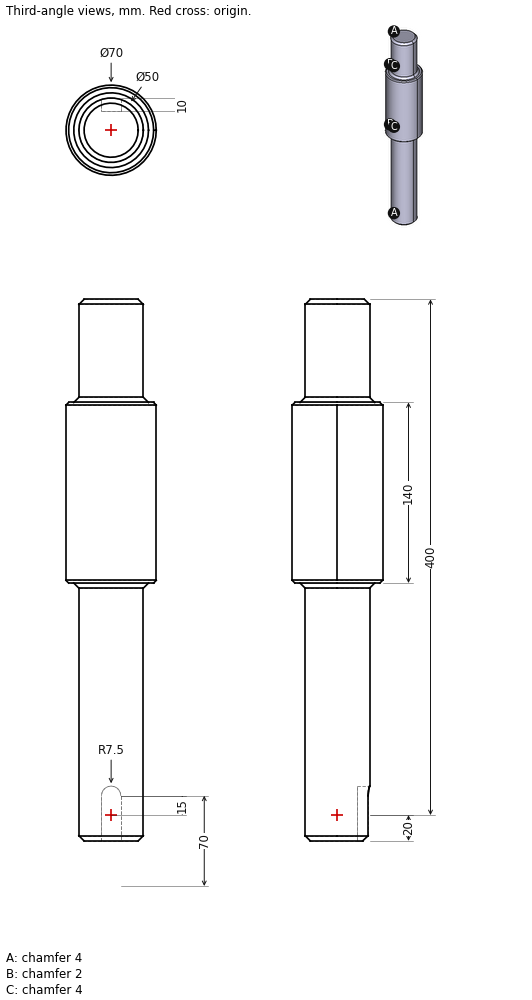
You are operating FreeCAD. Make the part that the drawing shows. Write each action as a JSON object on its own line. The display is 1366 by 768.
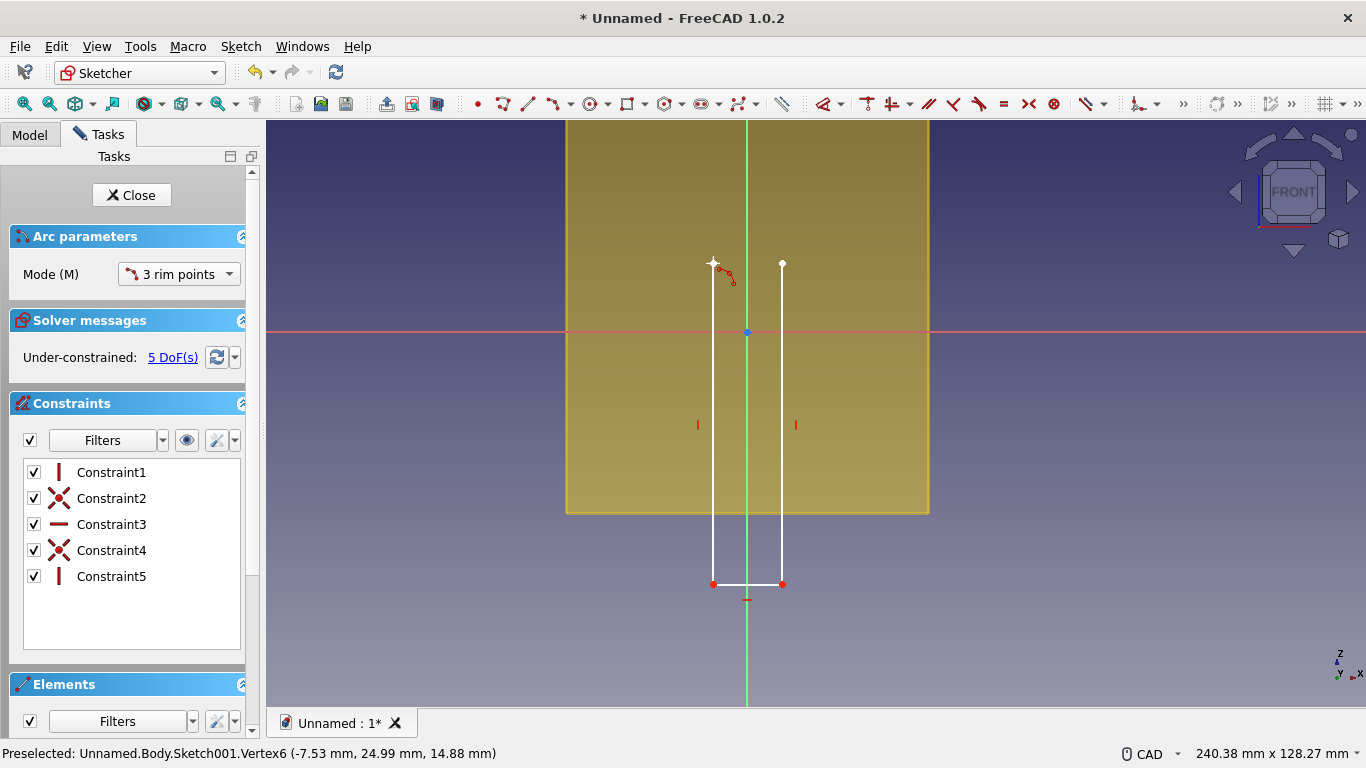
{"action": "left_click", "coordinate": [713, 264]}
{"action": "left_click", "coordinate": [782, 264]}
{"action": "left_click", "coordinate": [768, 236]}
{"action": "key", "text": "Escape"}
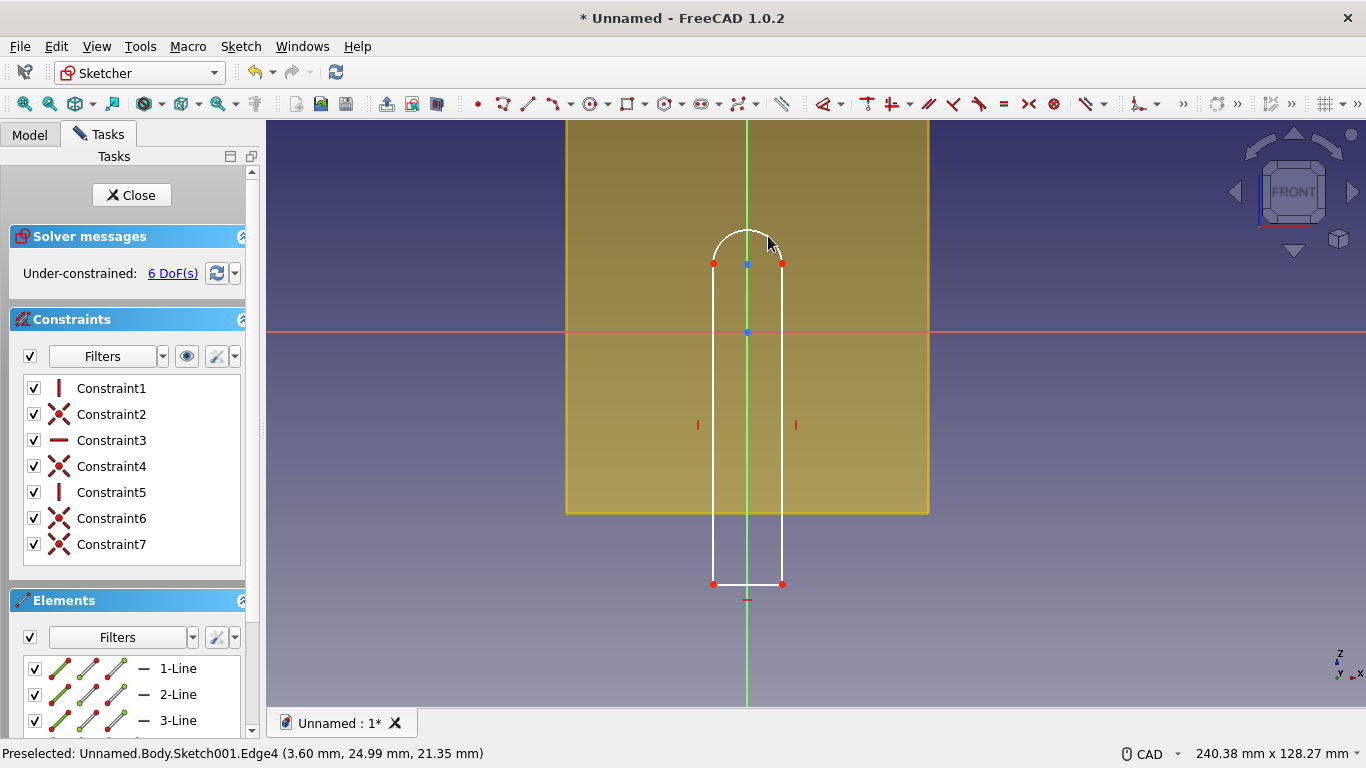
{"action": "left_click", "coordinate": [782, 360]}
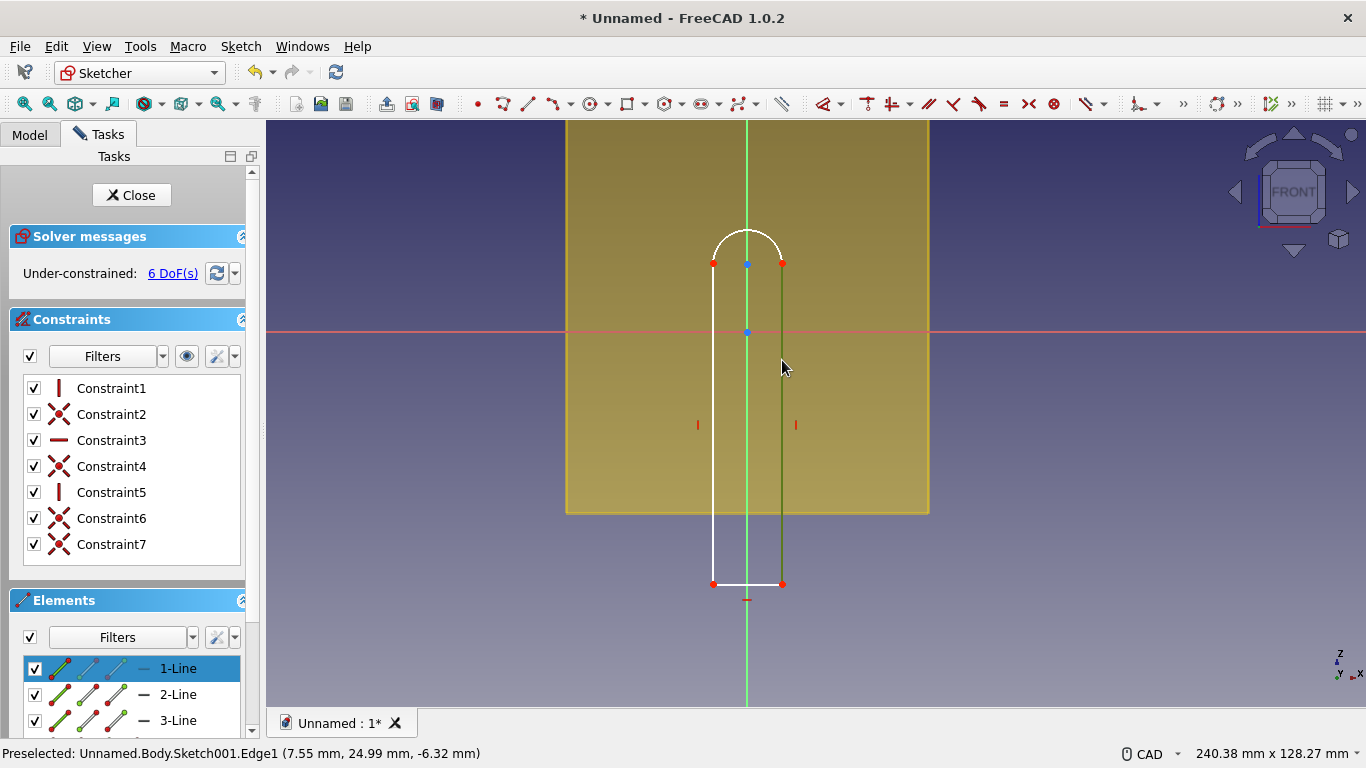
{"action": "left_click", "coordinate": [768, 237]}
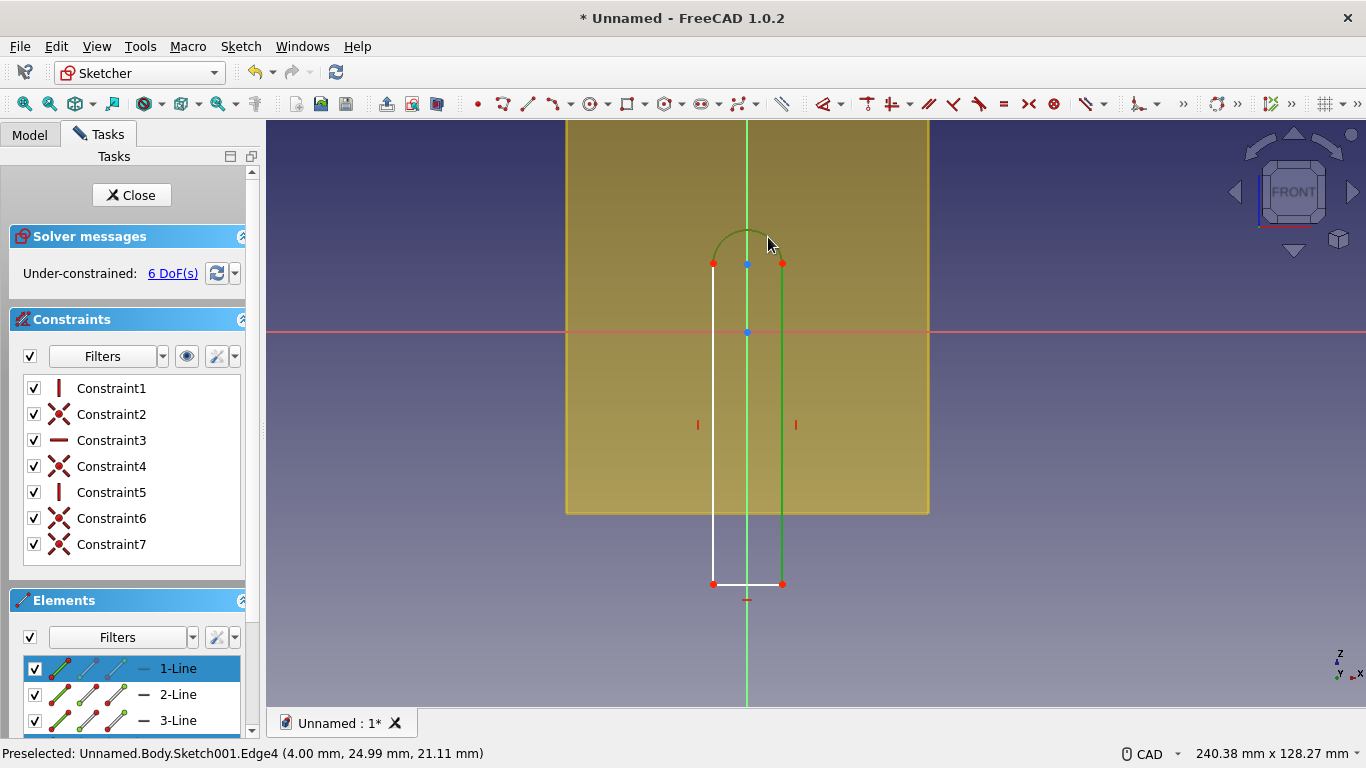
{"action": "left_click", "coordinate": [979, 104]}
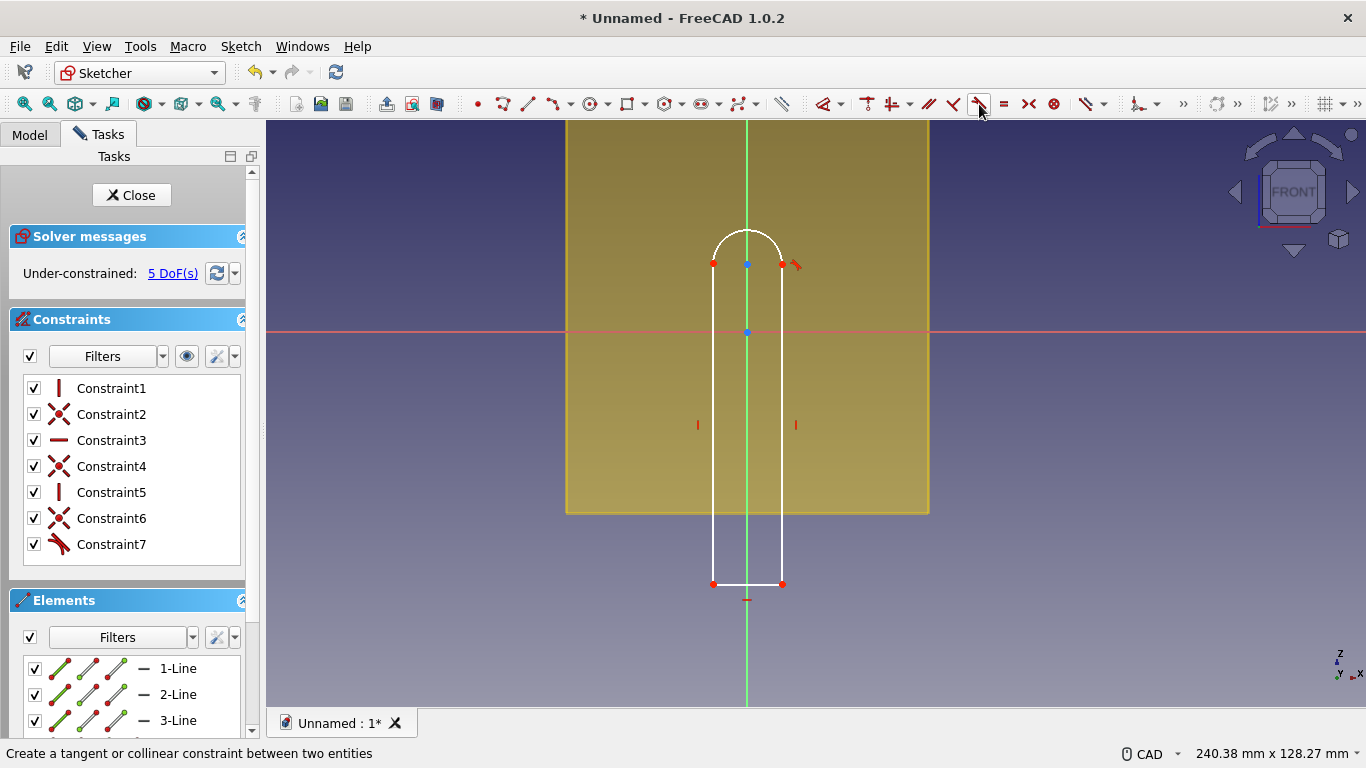
{"action": "left_click", "coordinate": [713, 489]}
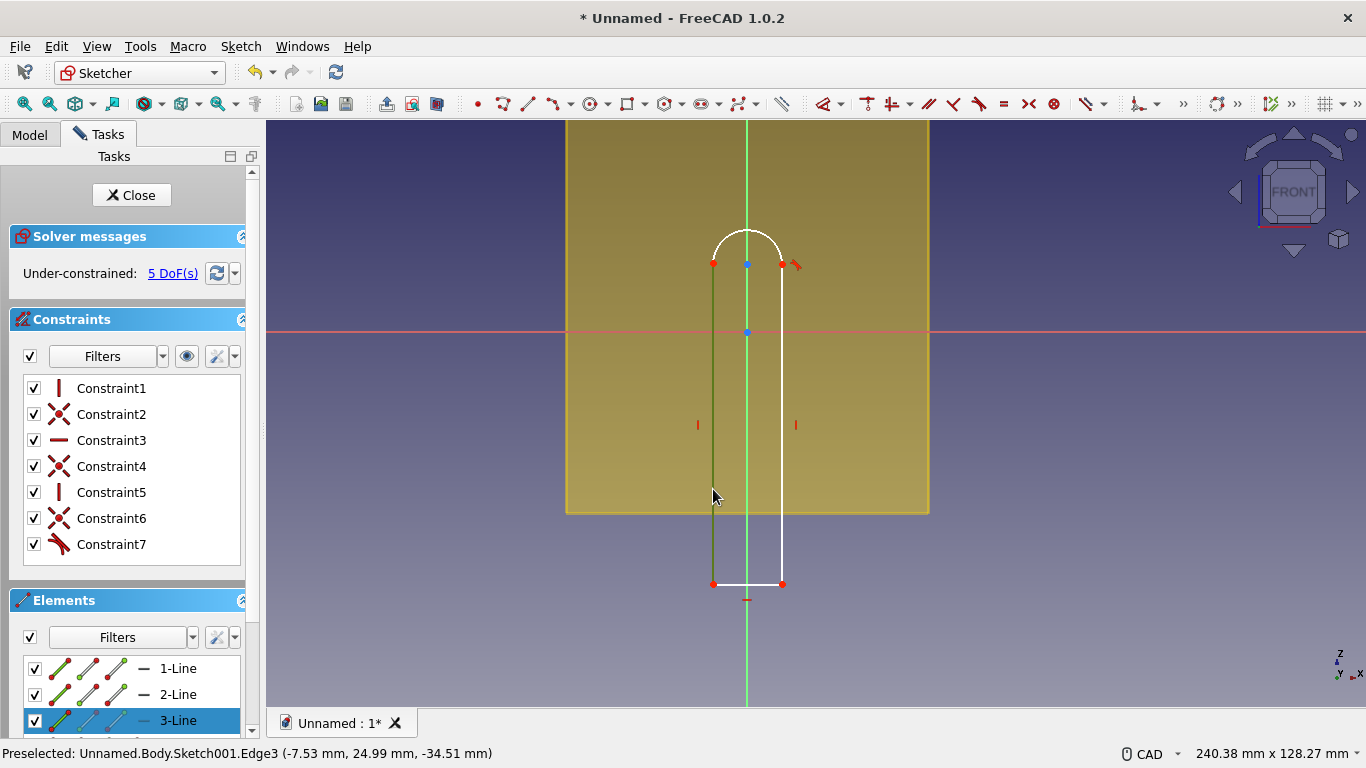
{"action": "left_click", "coordinate": [768, 237]}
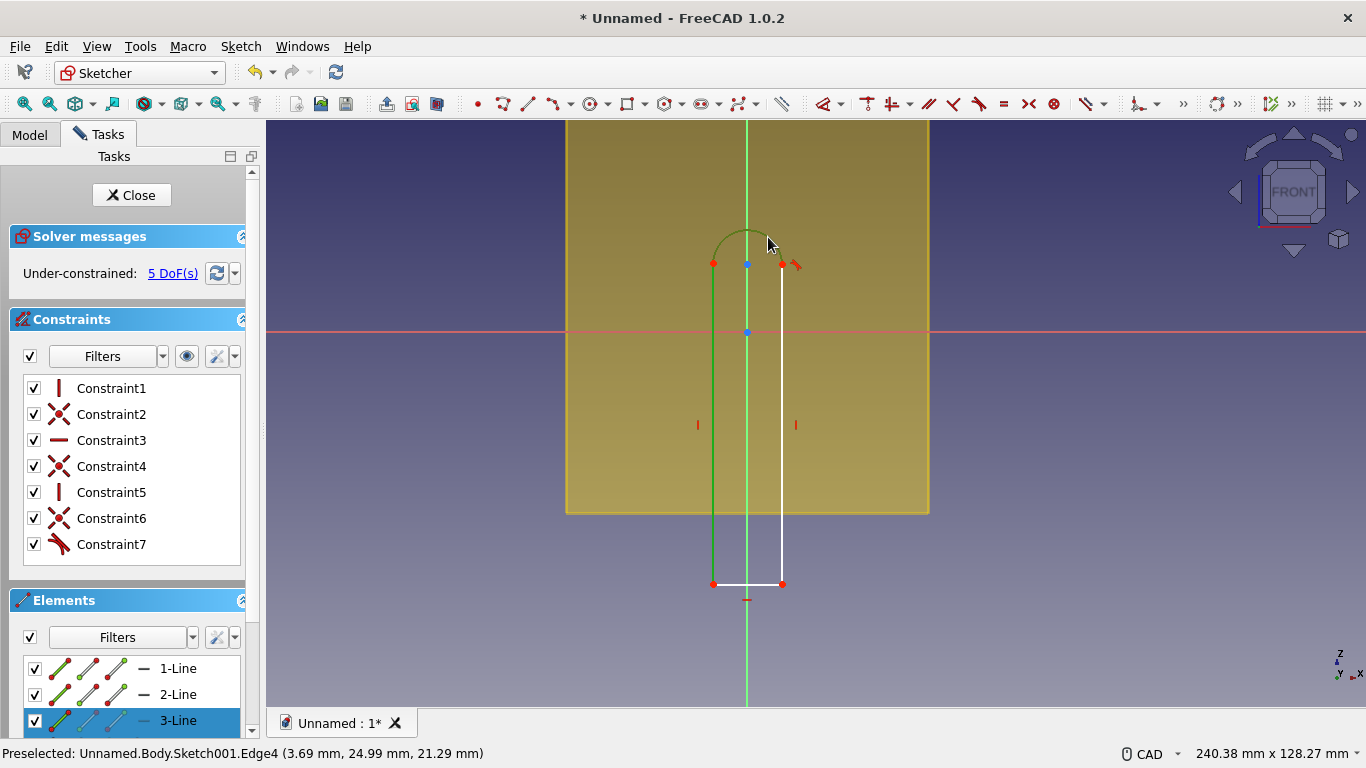
{"action": "left_click", "coordinate": [979, 104]}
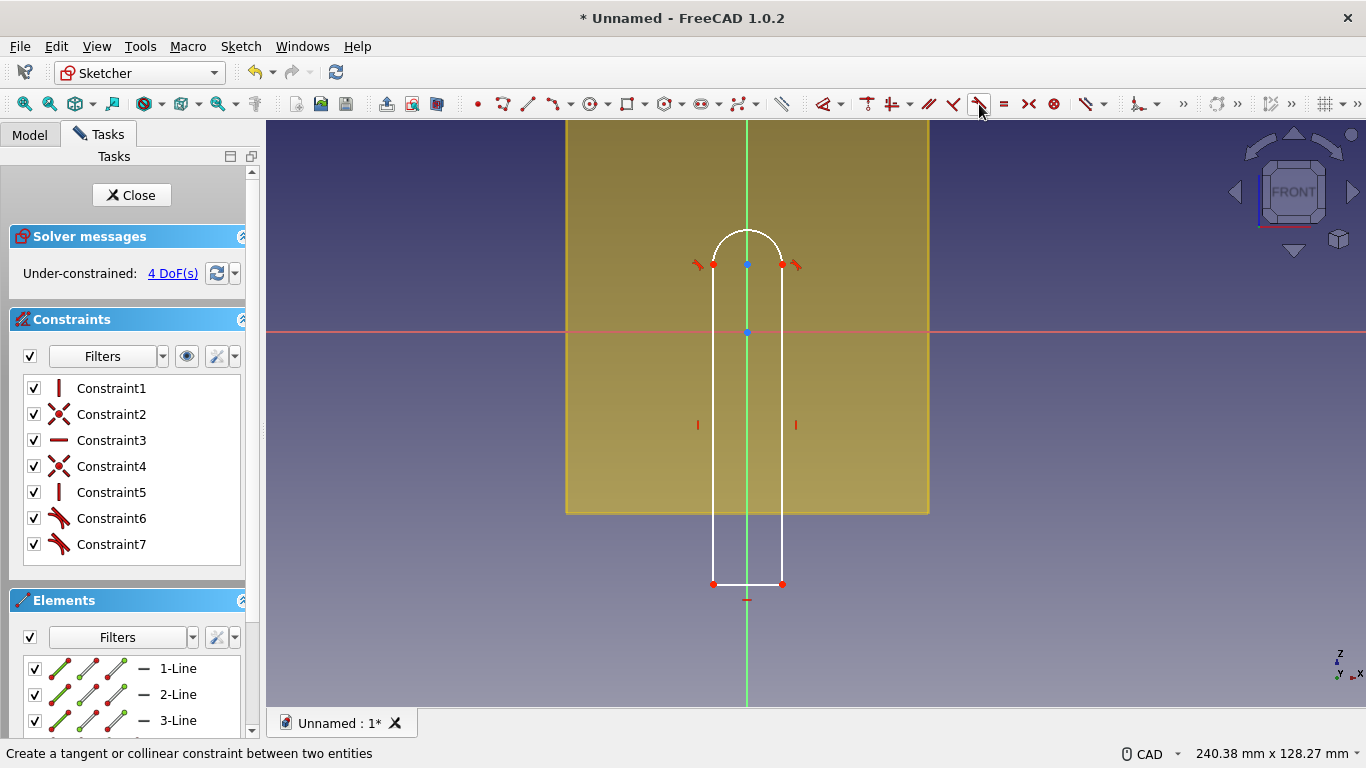
{"action": "left_click", "coordinate": [747, 265]}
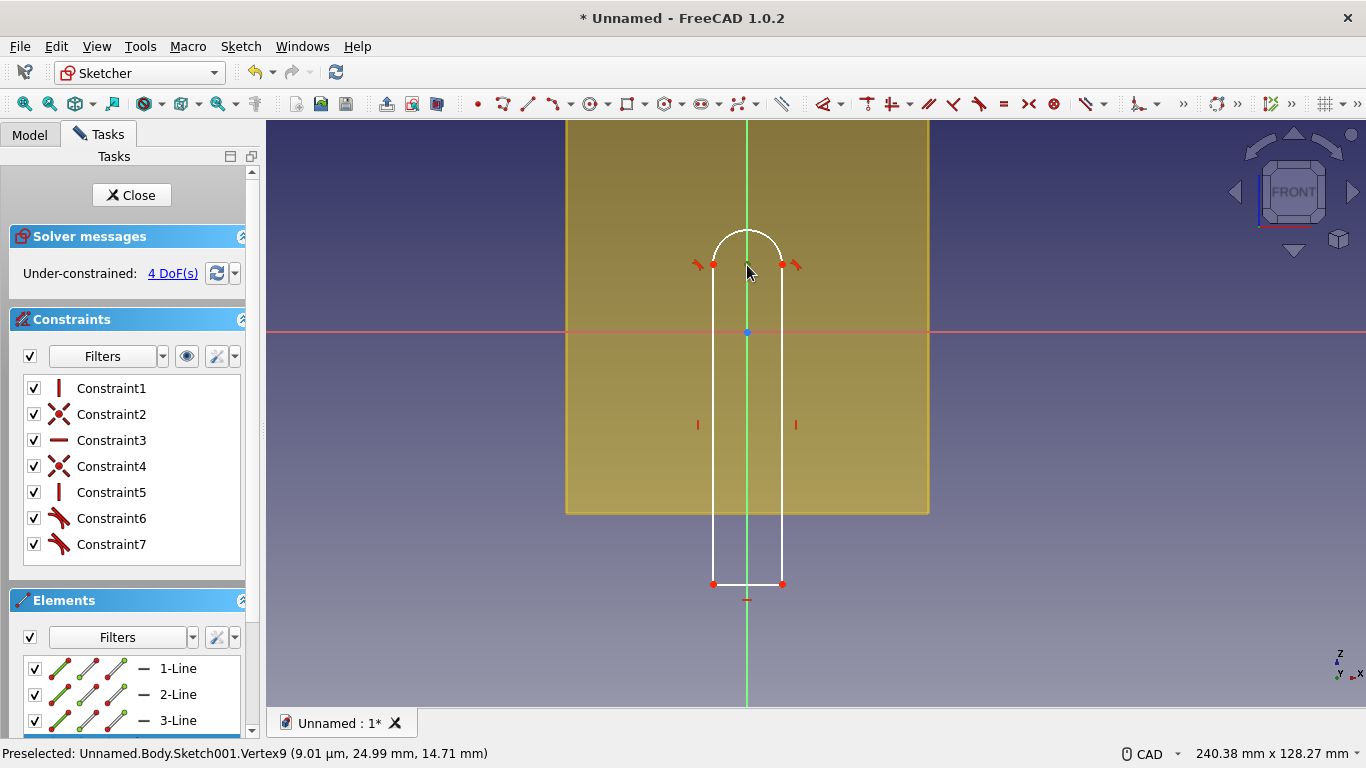
{"action": "left_click", "coordinate": [747, 641]}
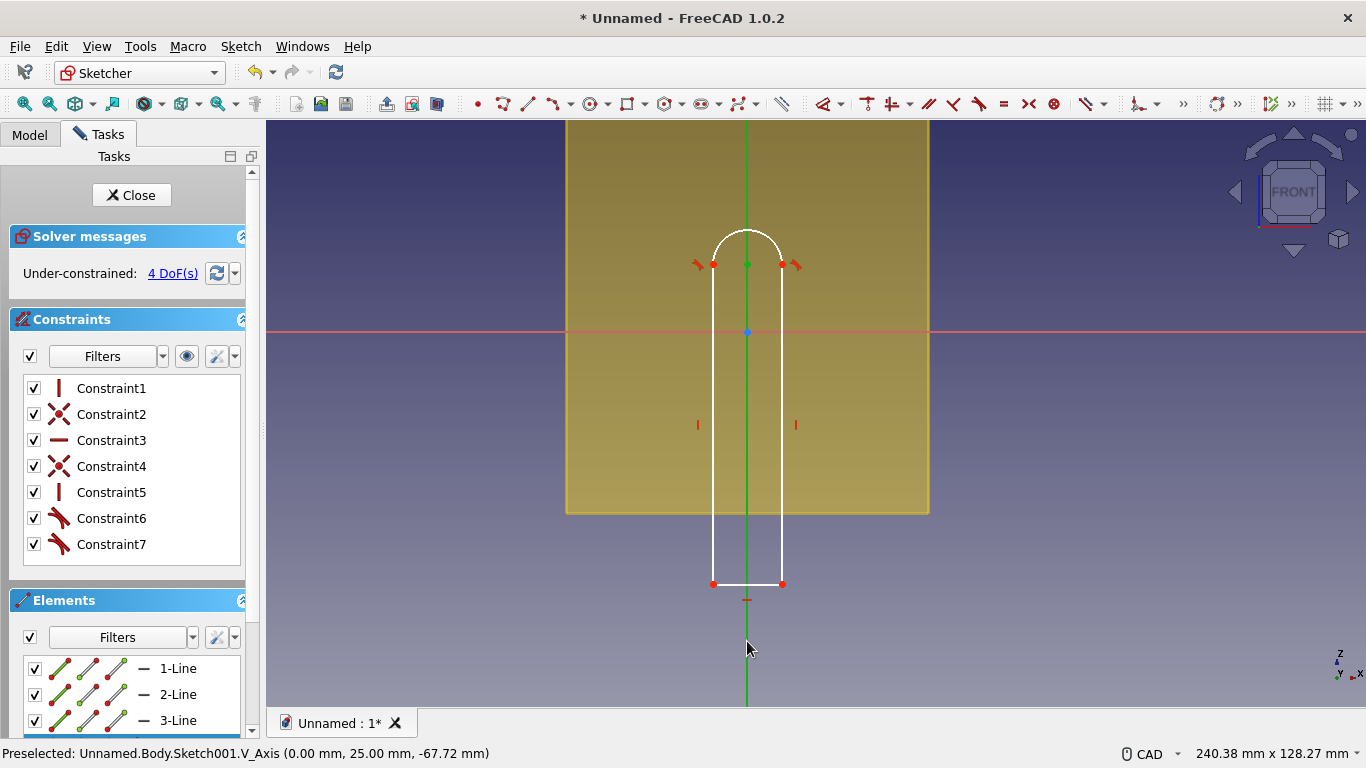
{"action": "left_click", "coordinate": [867, 104]}